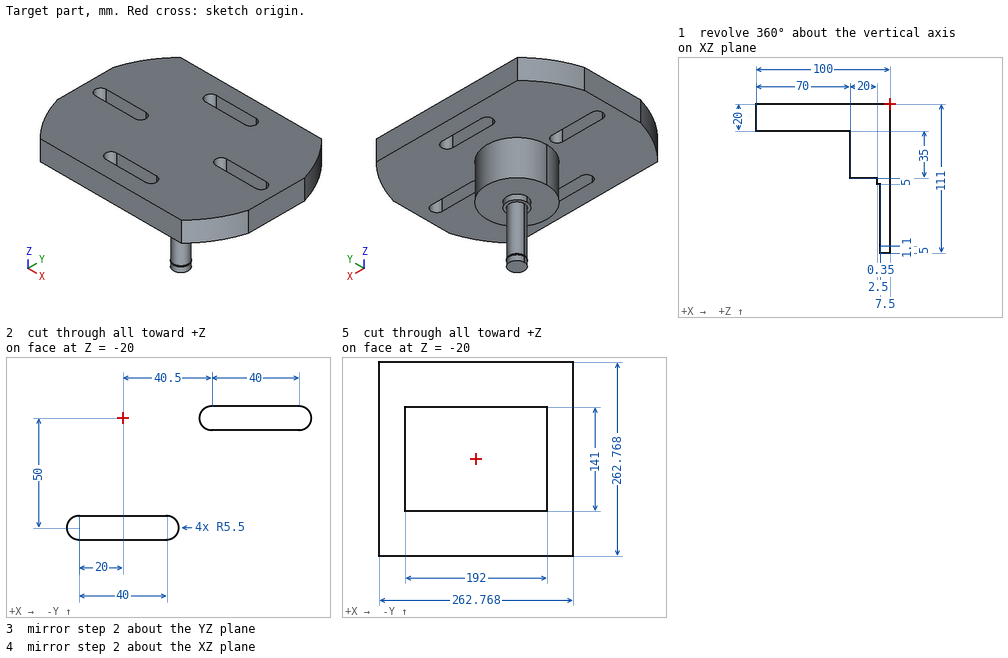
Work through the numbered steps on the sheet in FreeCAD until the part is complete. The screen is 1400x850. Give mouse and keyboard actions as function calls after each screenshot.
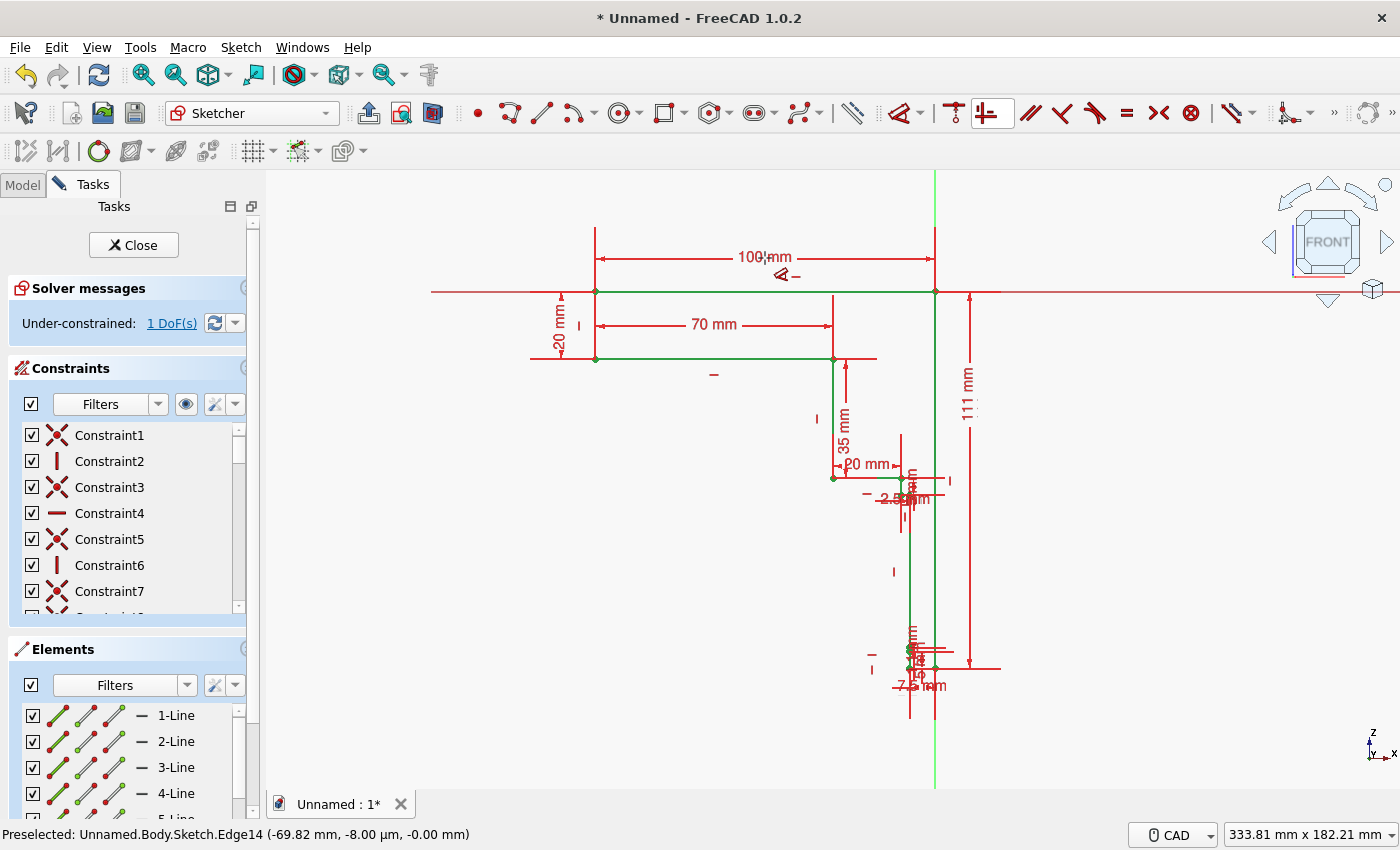
scroll(910, 652, up, 18)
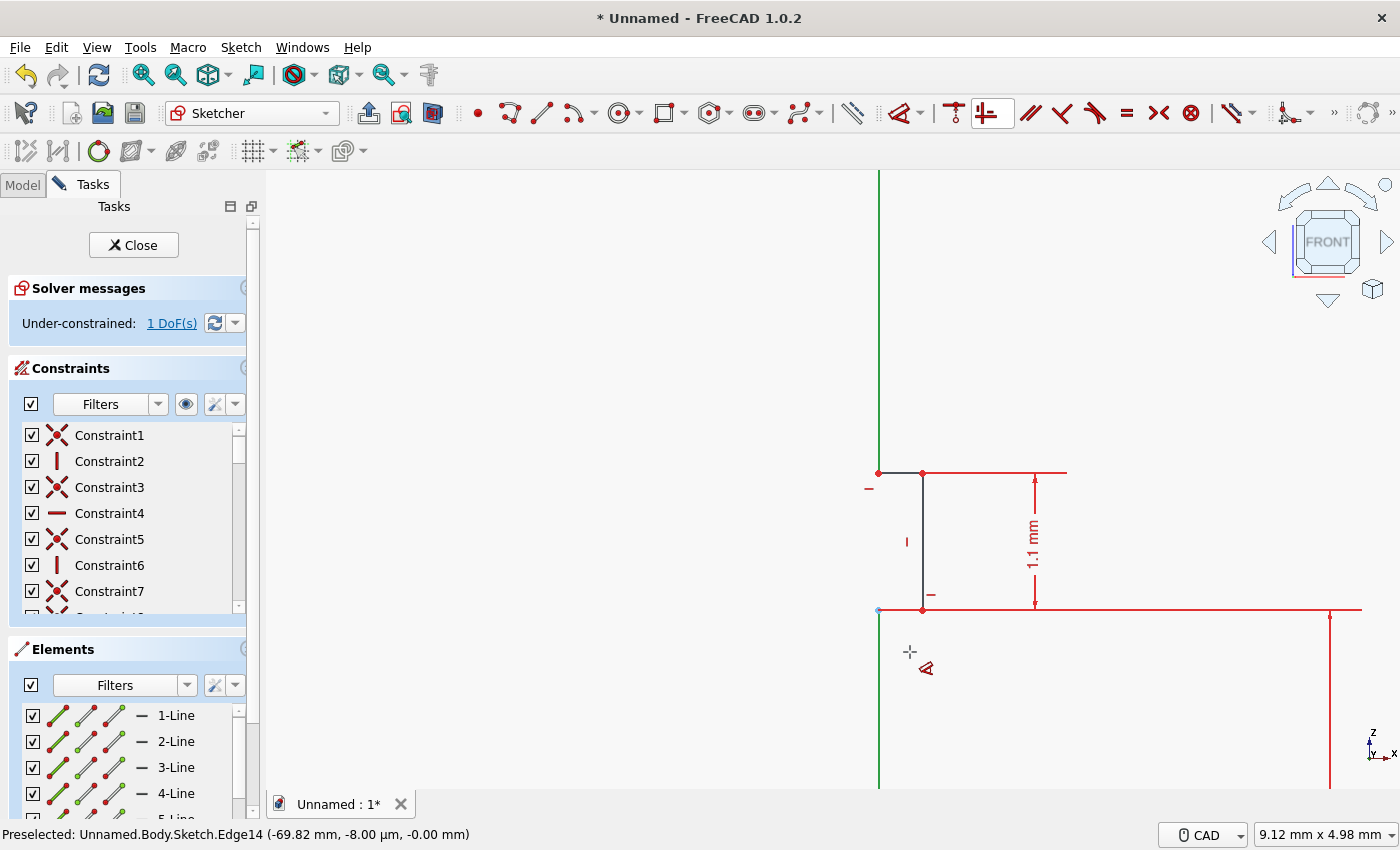
click(901, 610)
click(901, 644)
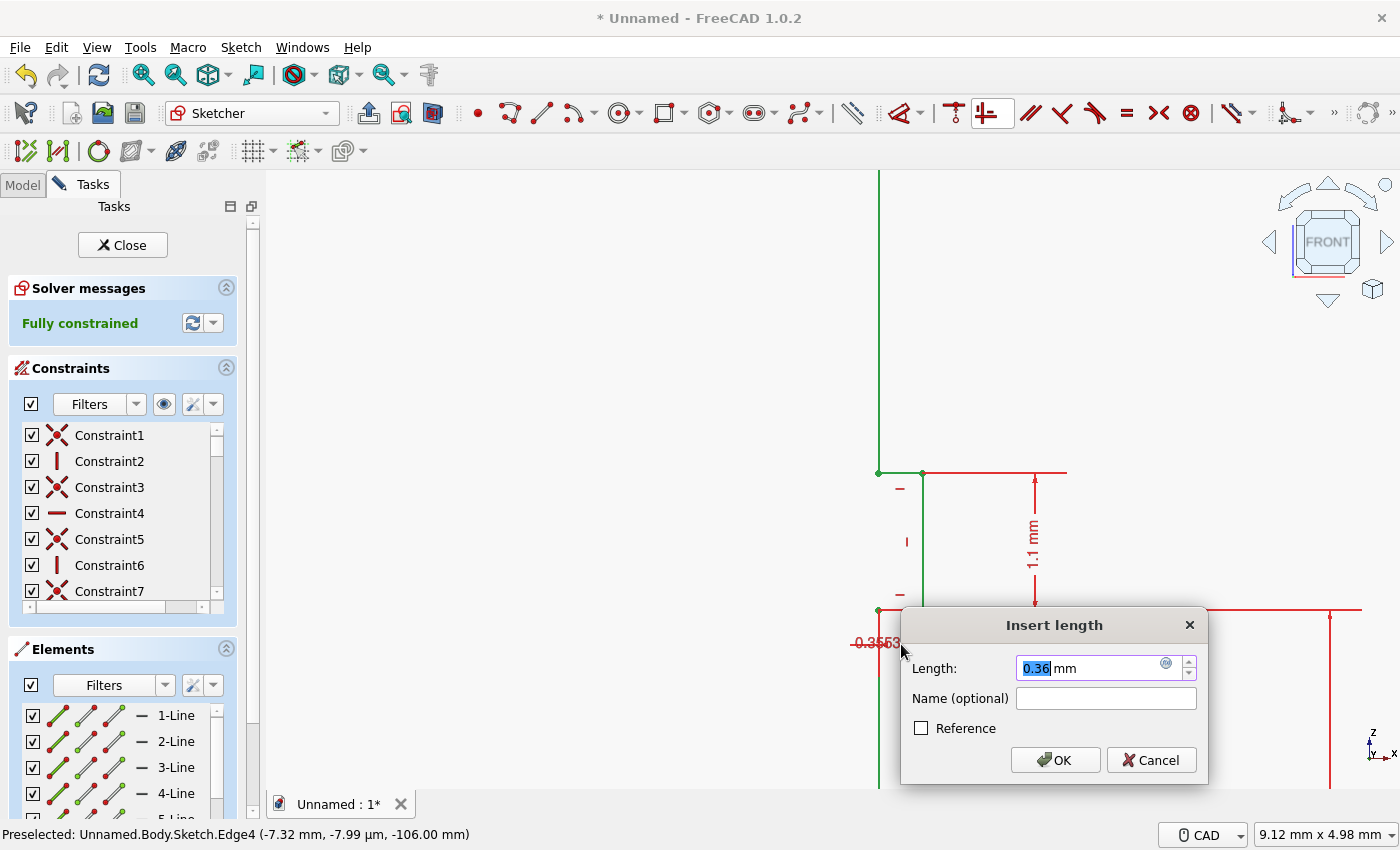
text(0.35)
key(Return)
key(Escape)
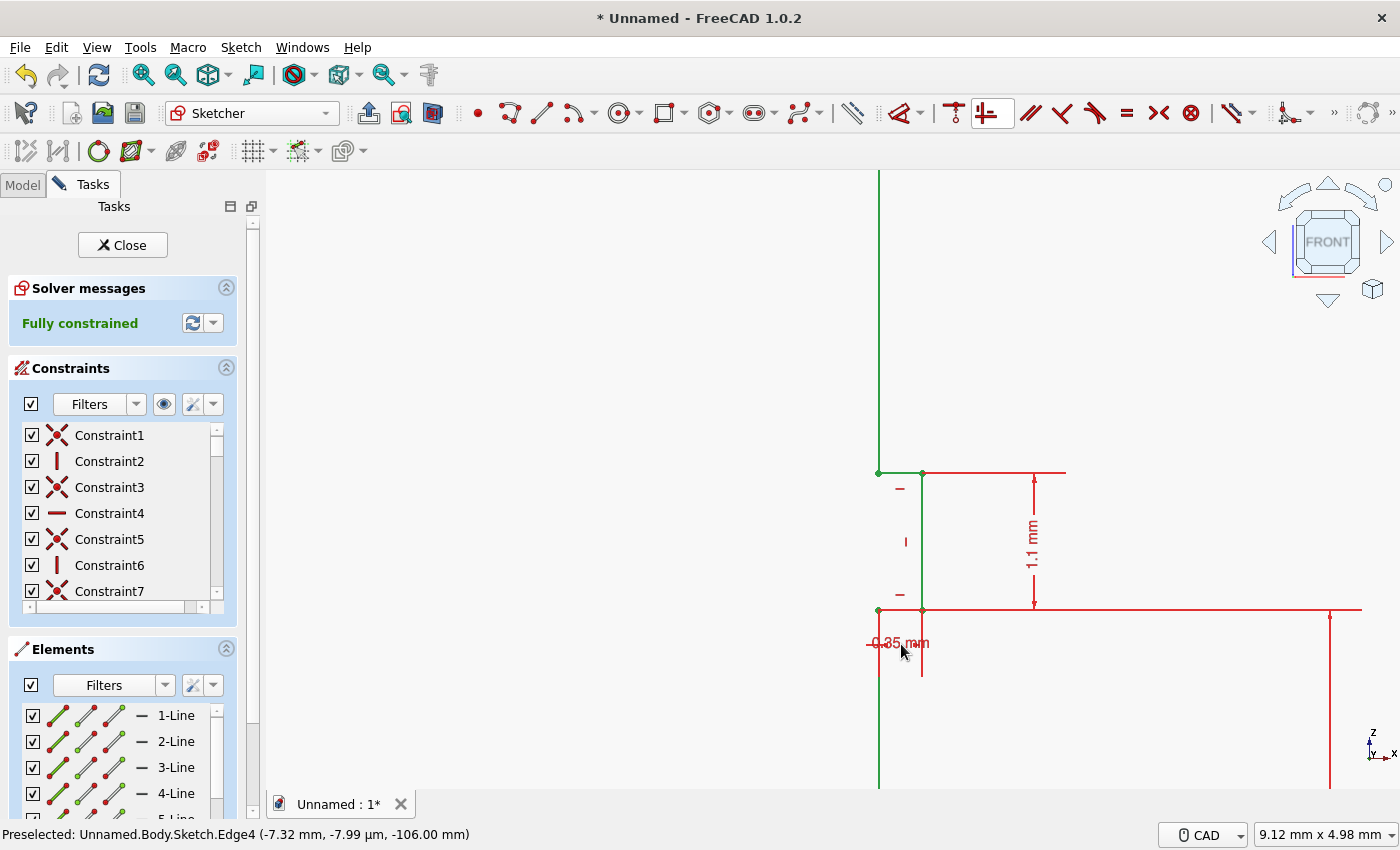
click(123, 245)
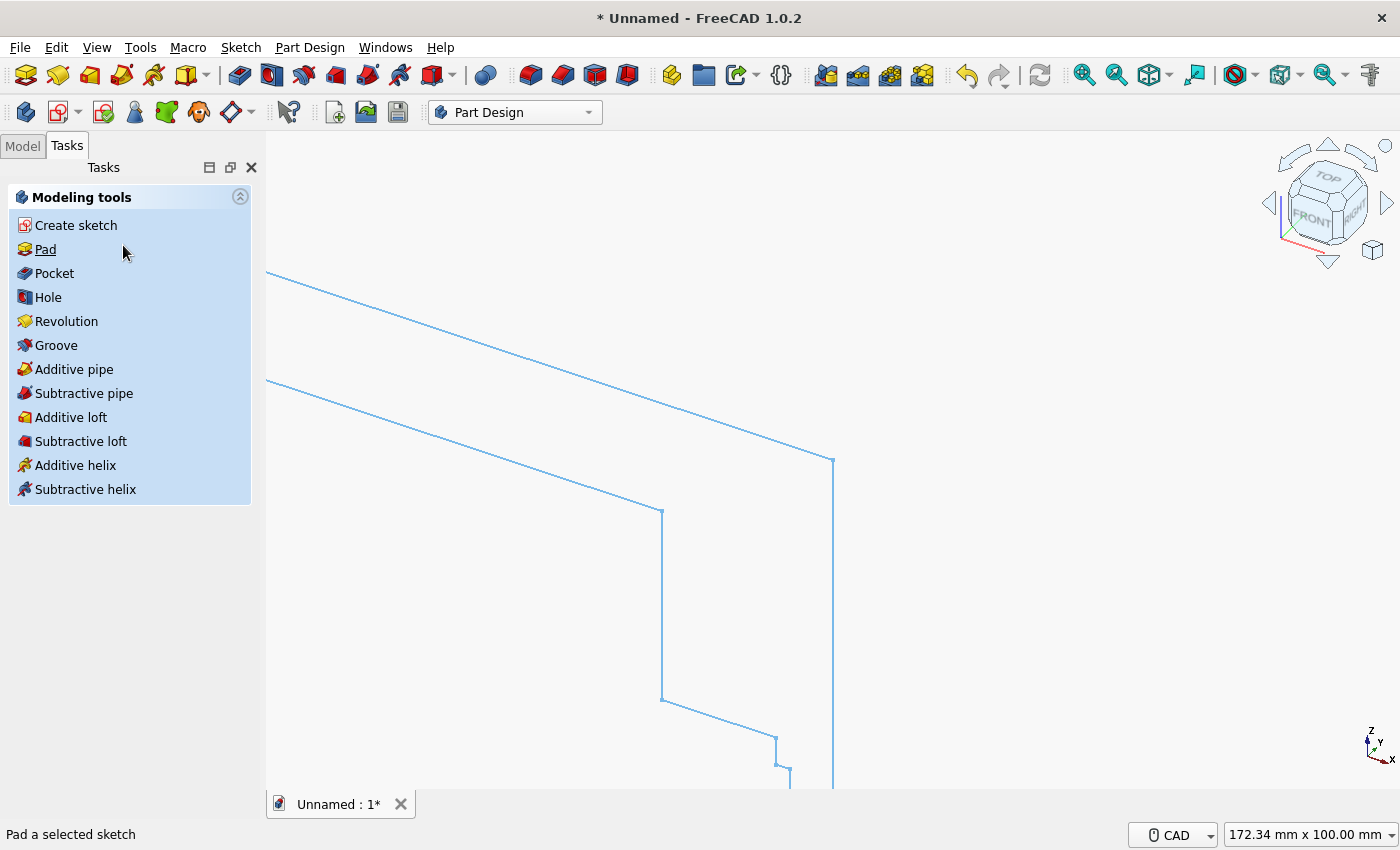
click(58, 76)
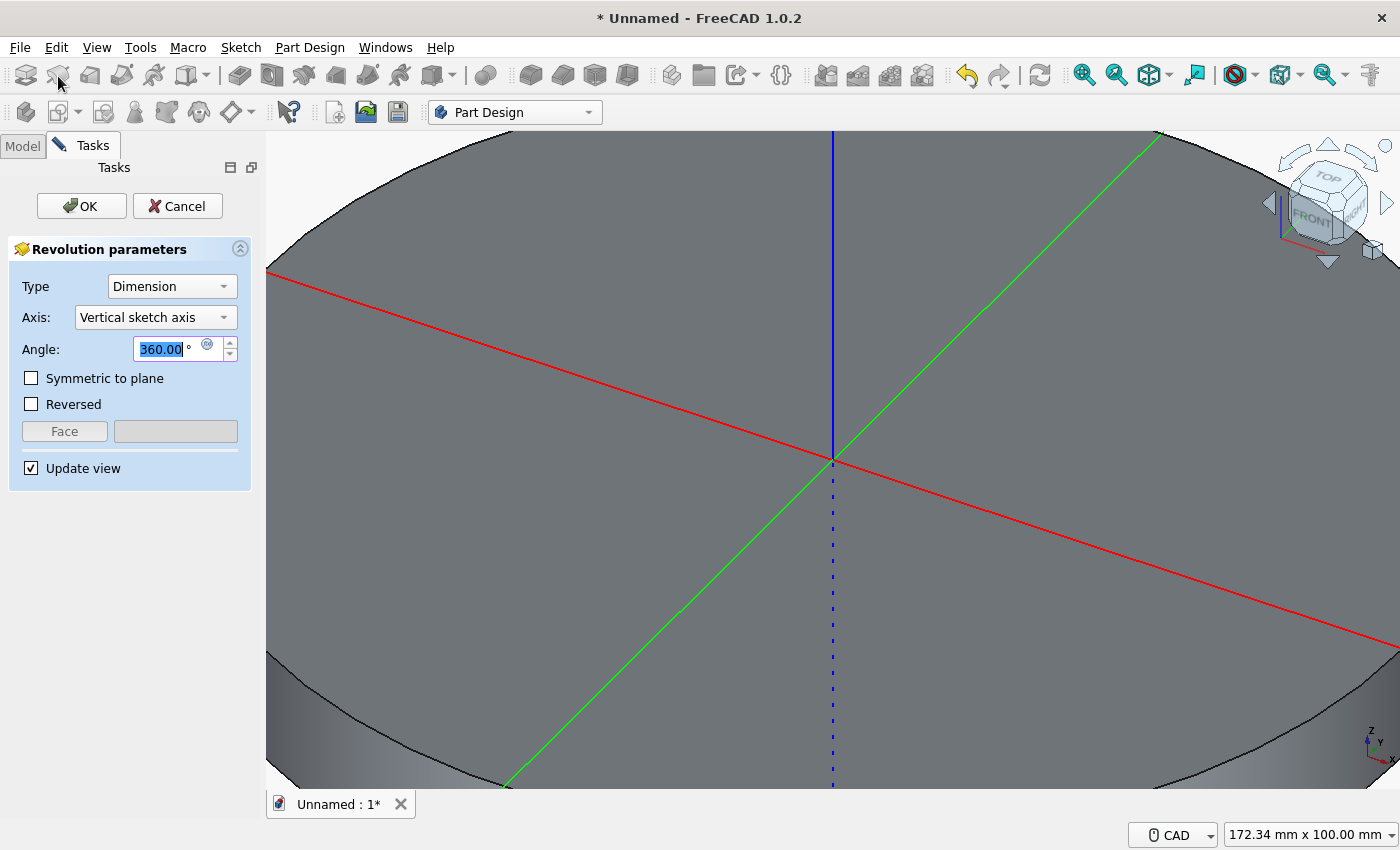
click(82, 206)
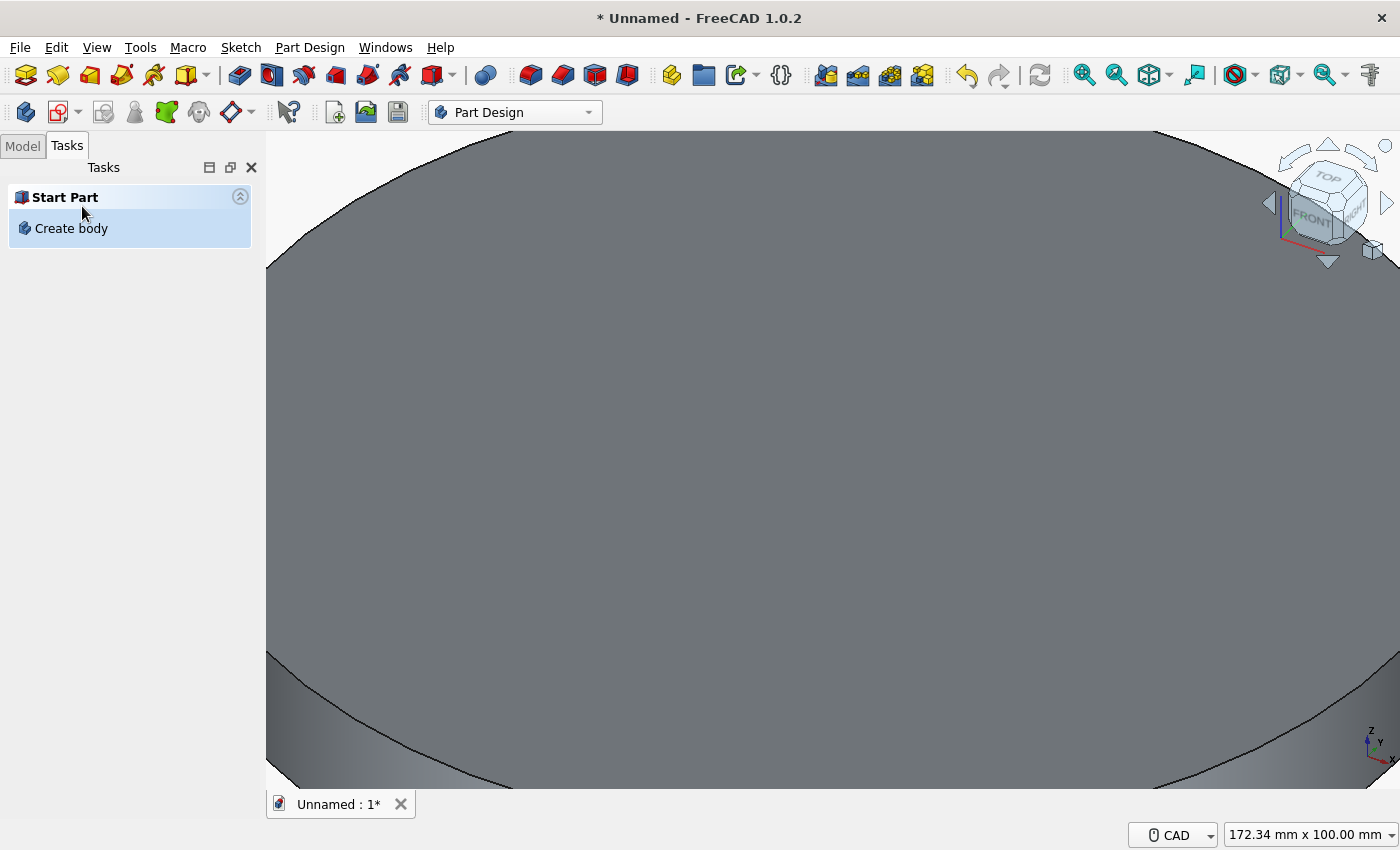
click(1086, 76)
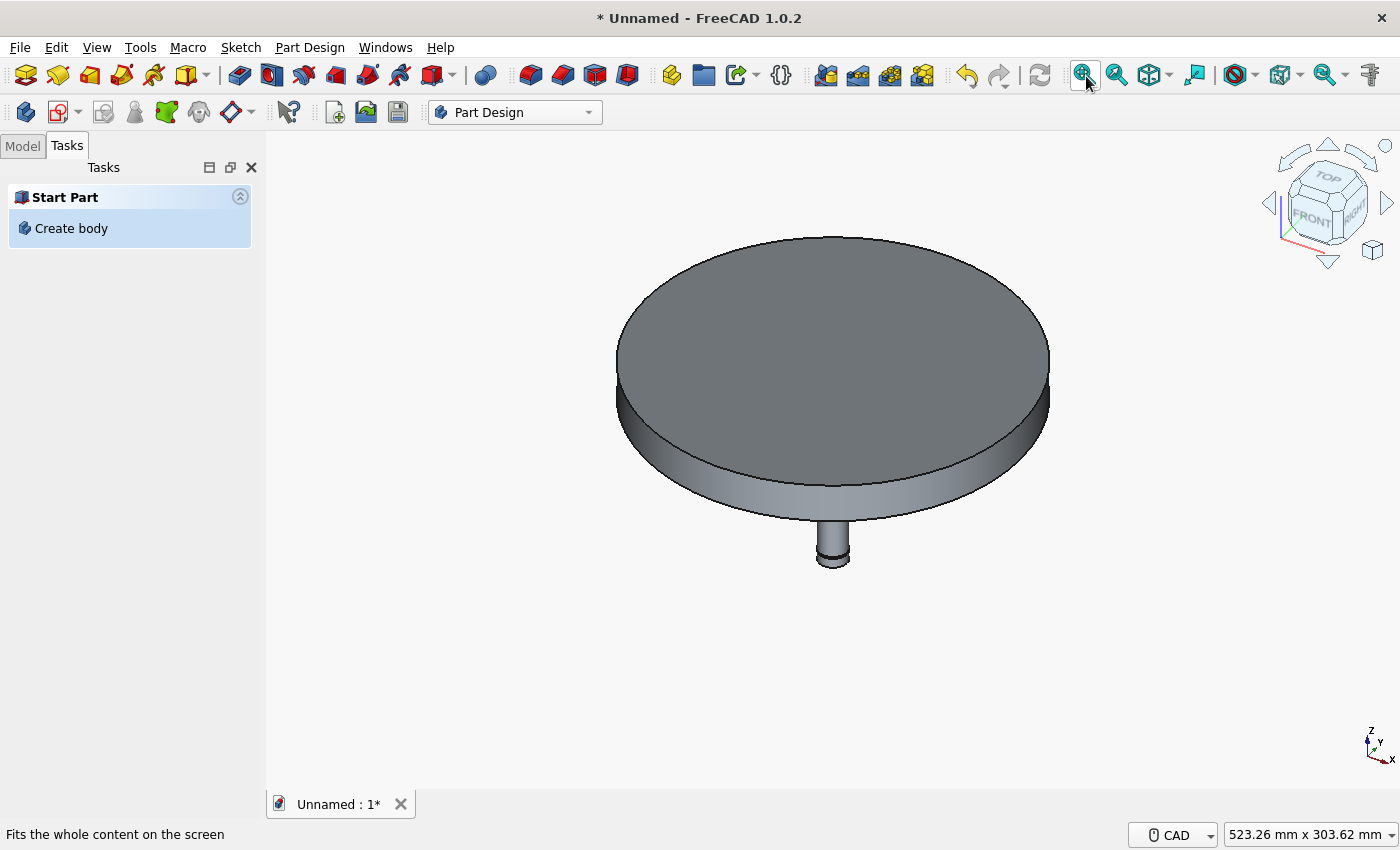
key(5)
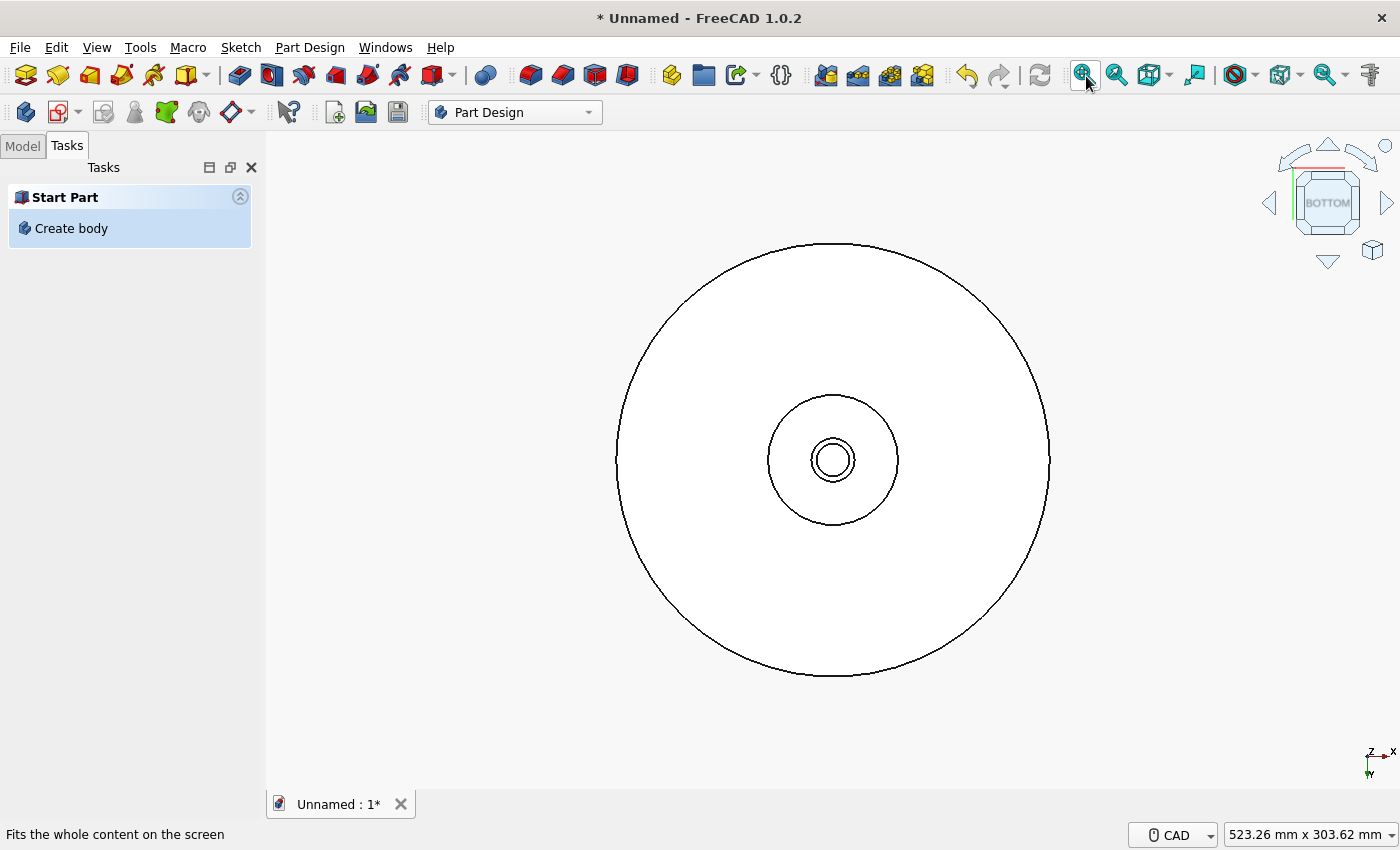
click(895, 583)